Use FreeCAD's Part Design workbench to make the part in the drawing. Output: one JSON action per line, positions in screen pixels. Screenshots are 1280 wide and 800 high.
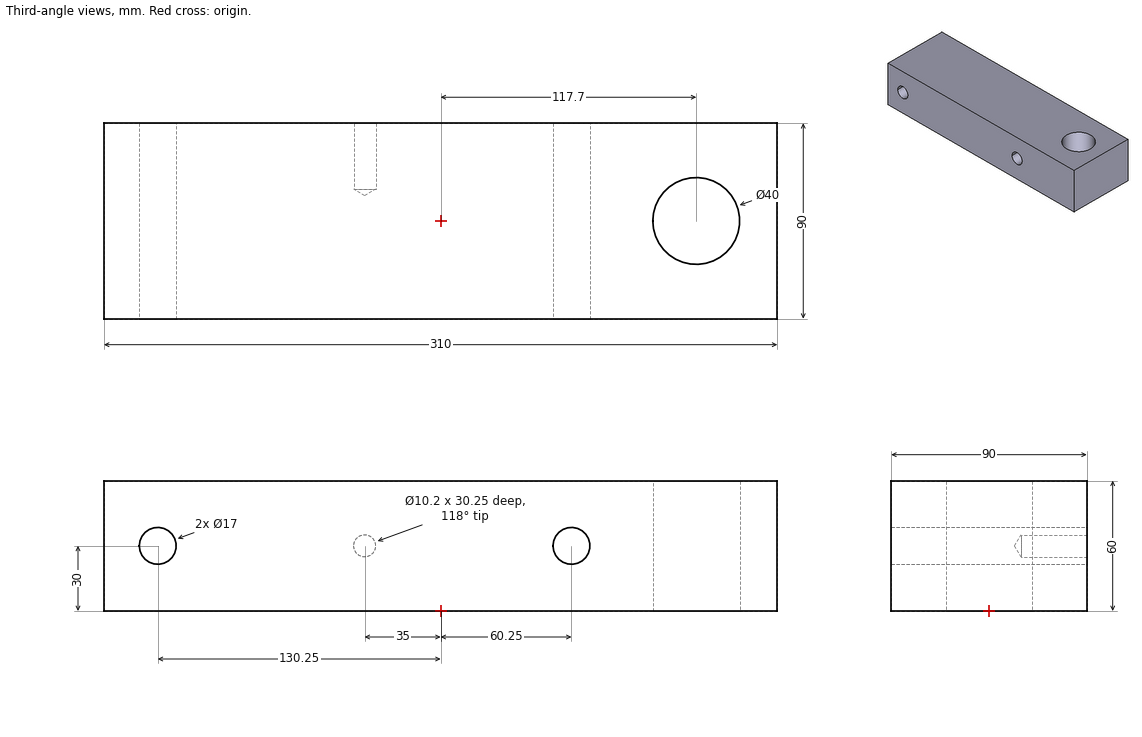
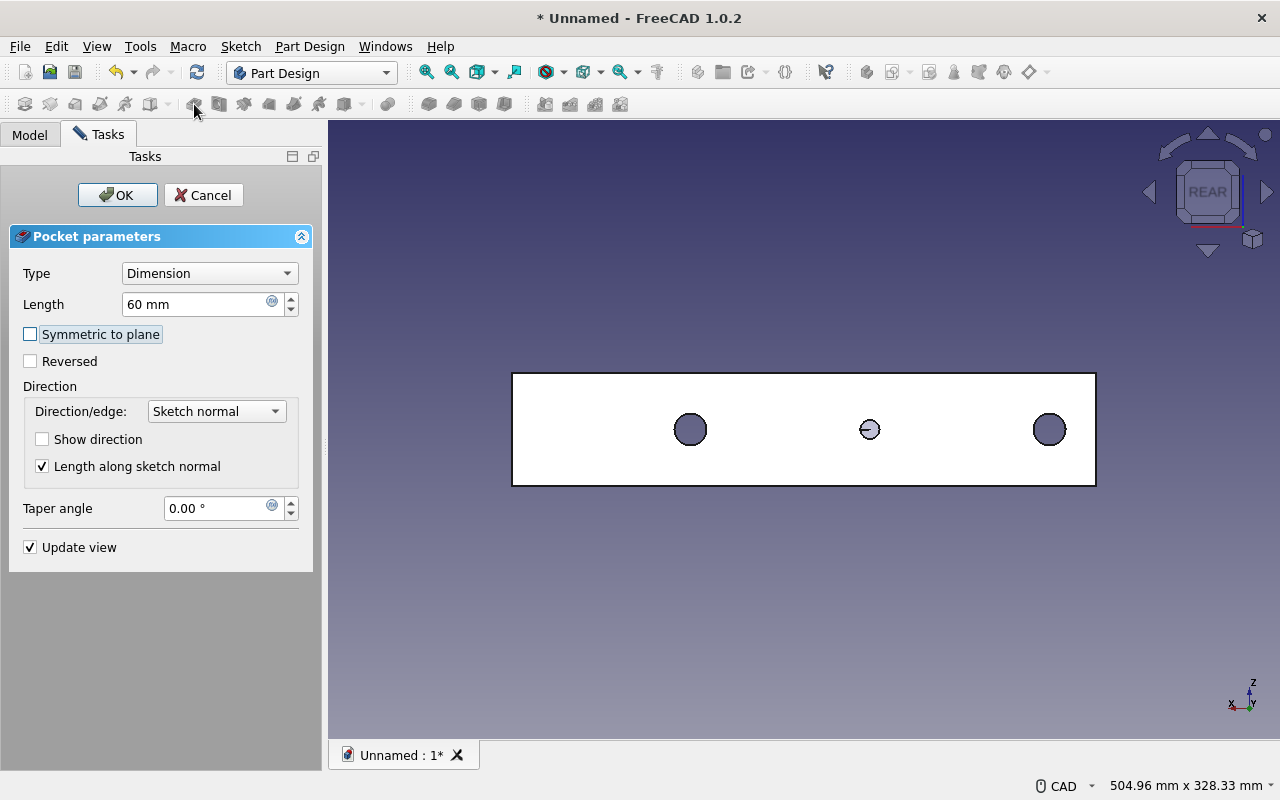
{"action": "left_click", "coordinate": [31, 361]}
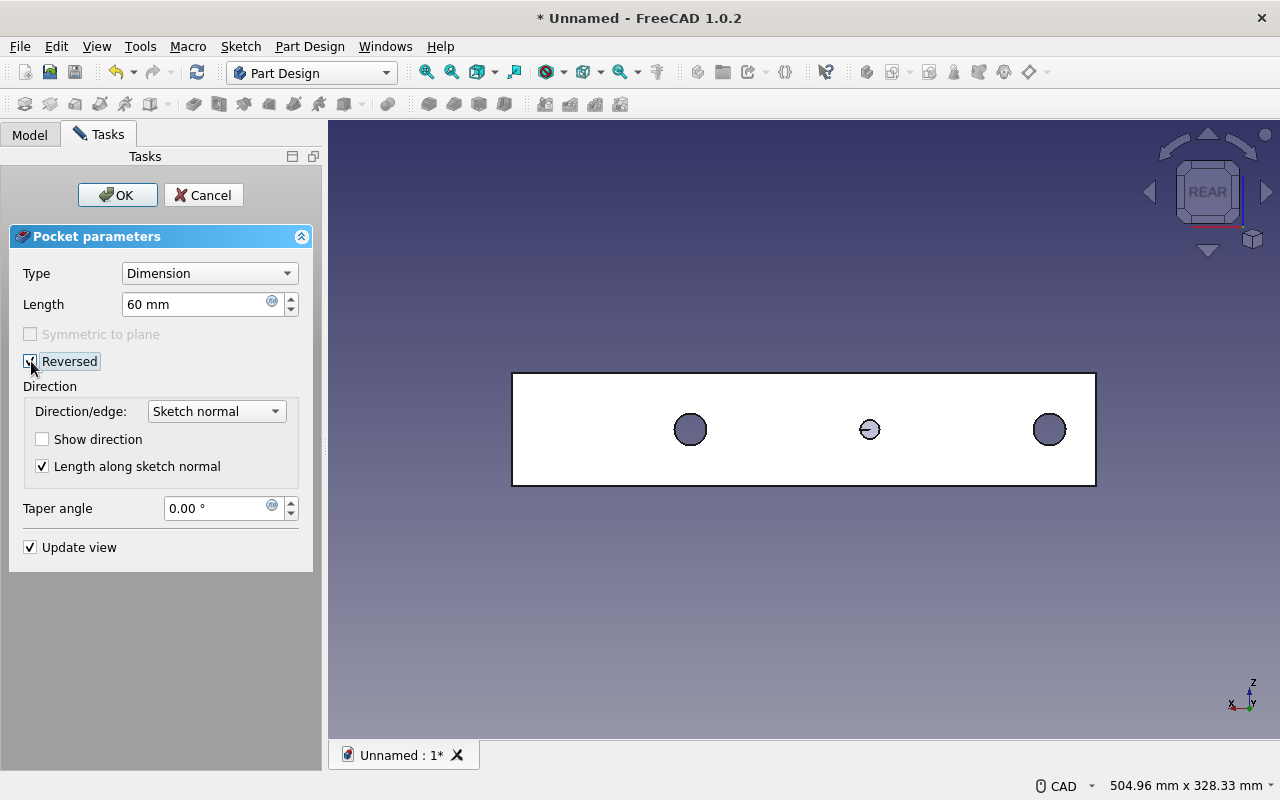
{"action": "left_click", "coordinate": [118, 195]}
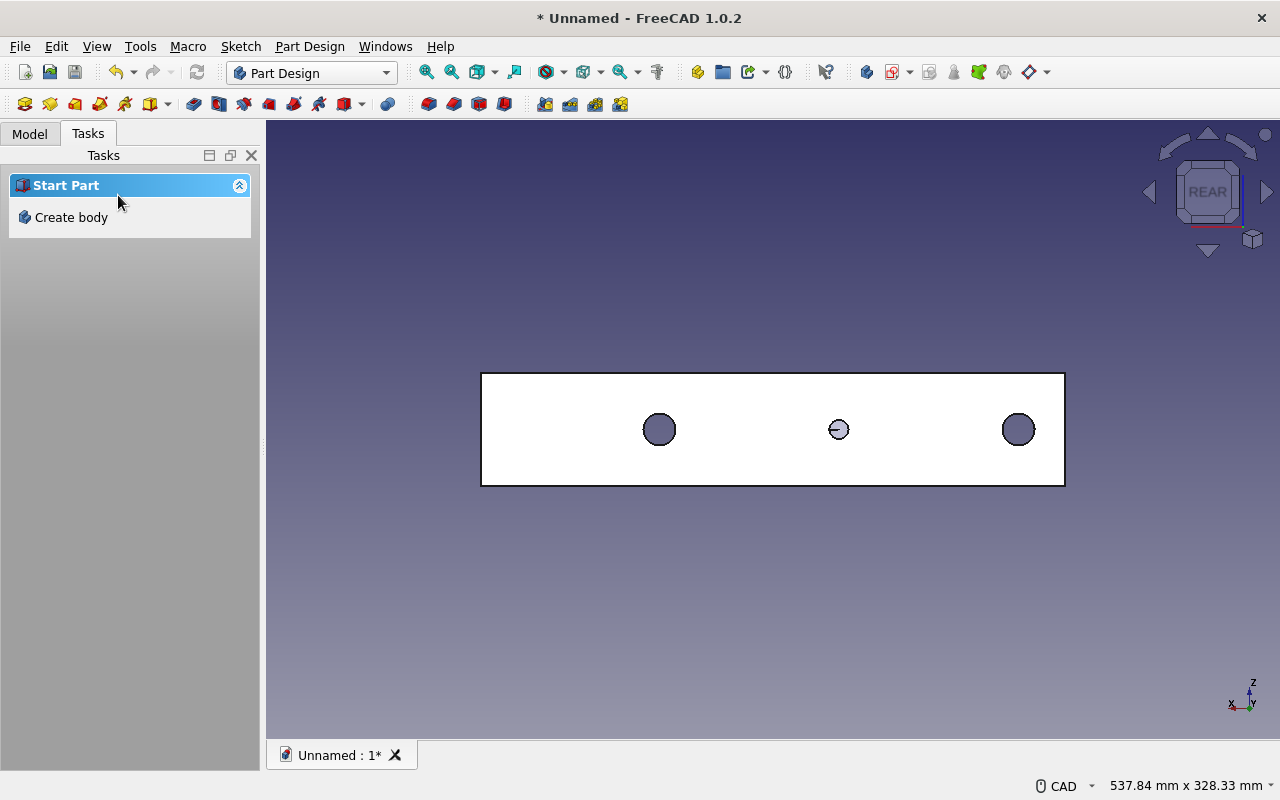
{"action": "key", "text": "0"}